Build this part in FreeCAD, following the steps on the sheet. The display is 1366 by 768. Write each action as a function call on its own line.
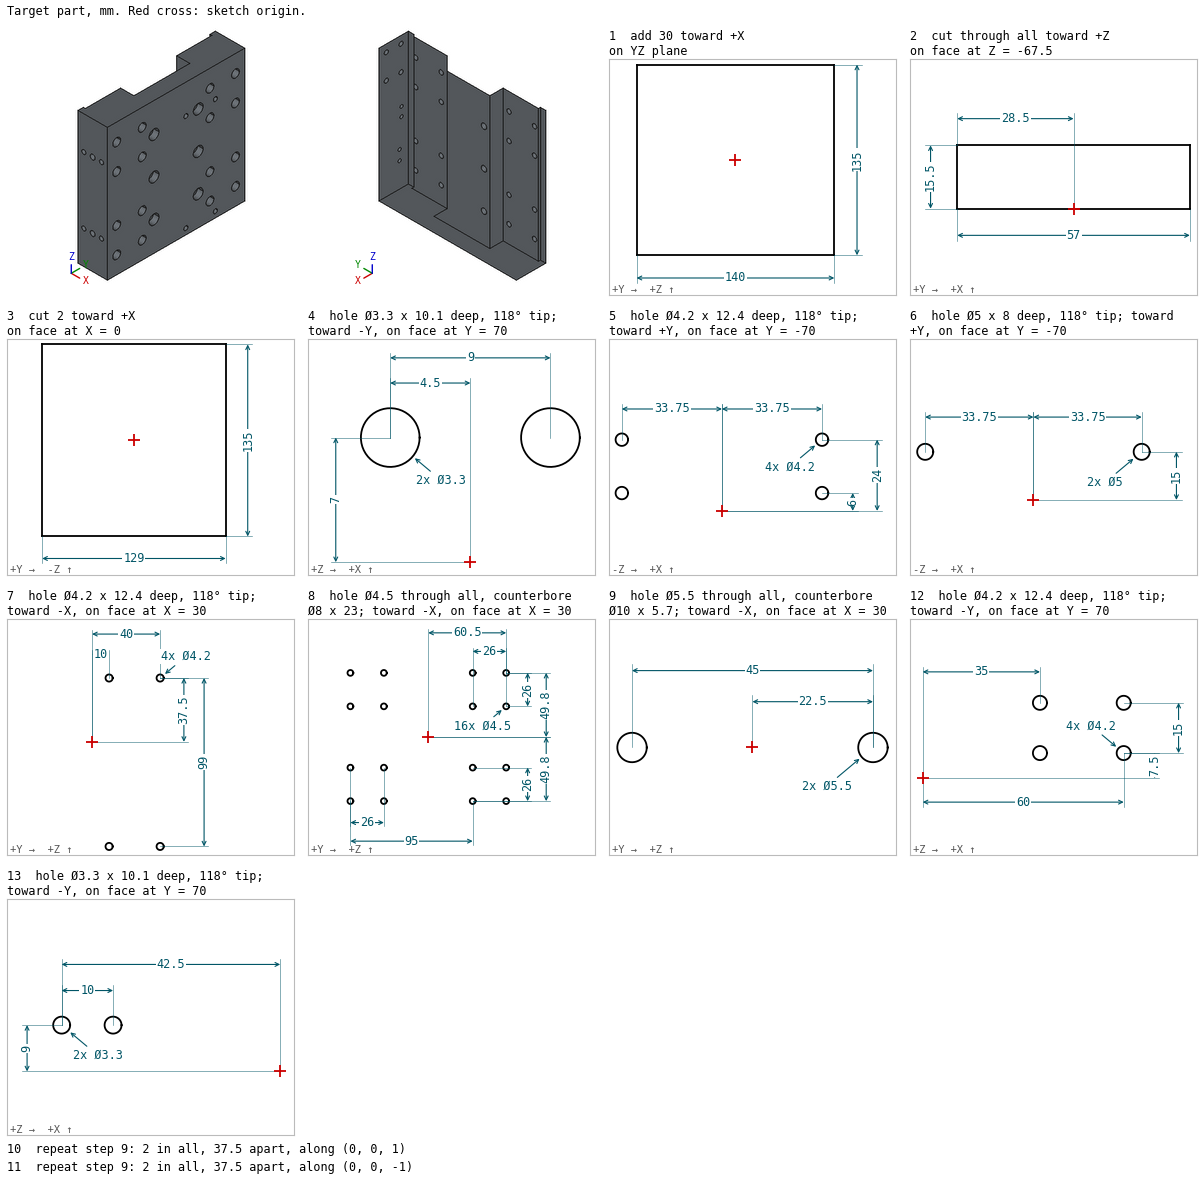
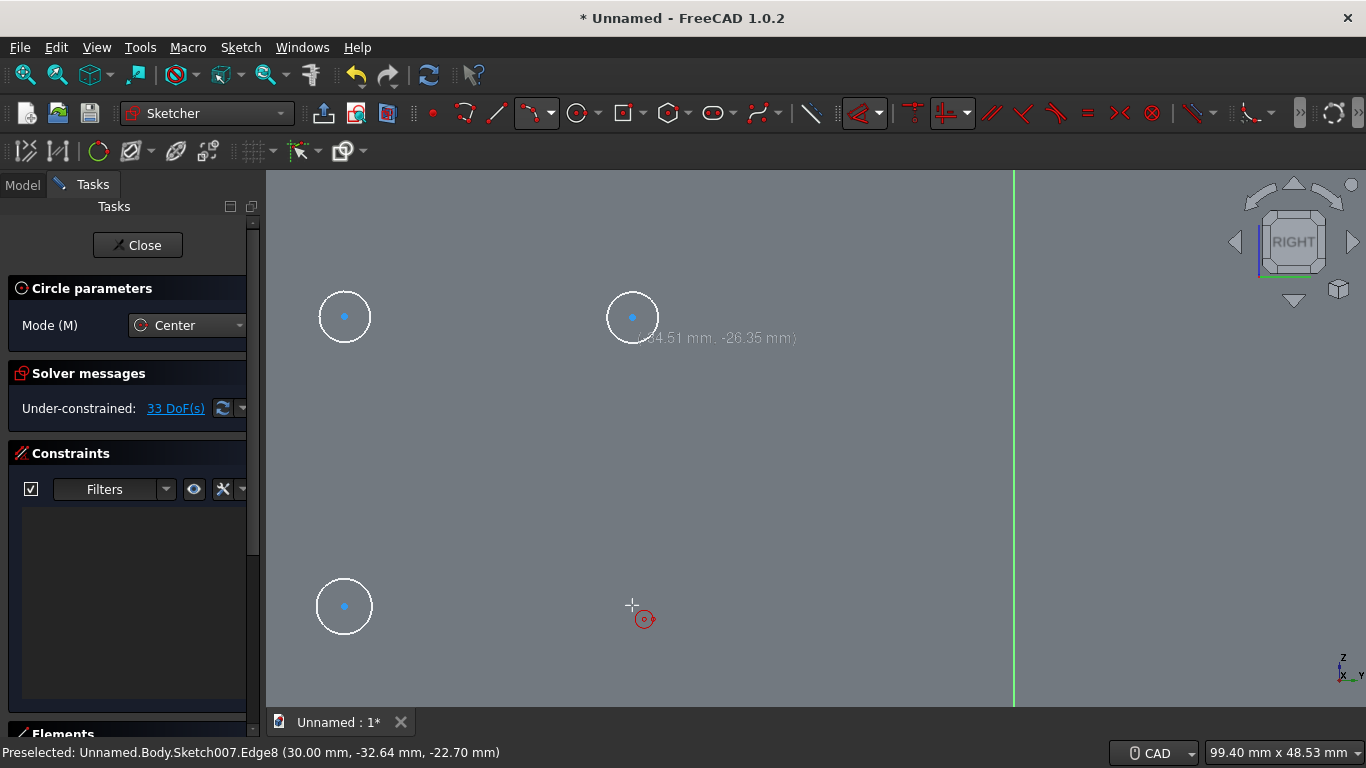
scroll(632, 605, down, 6)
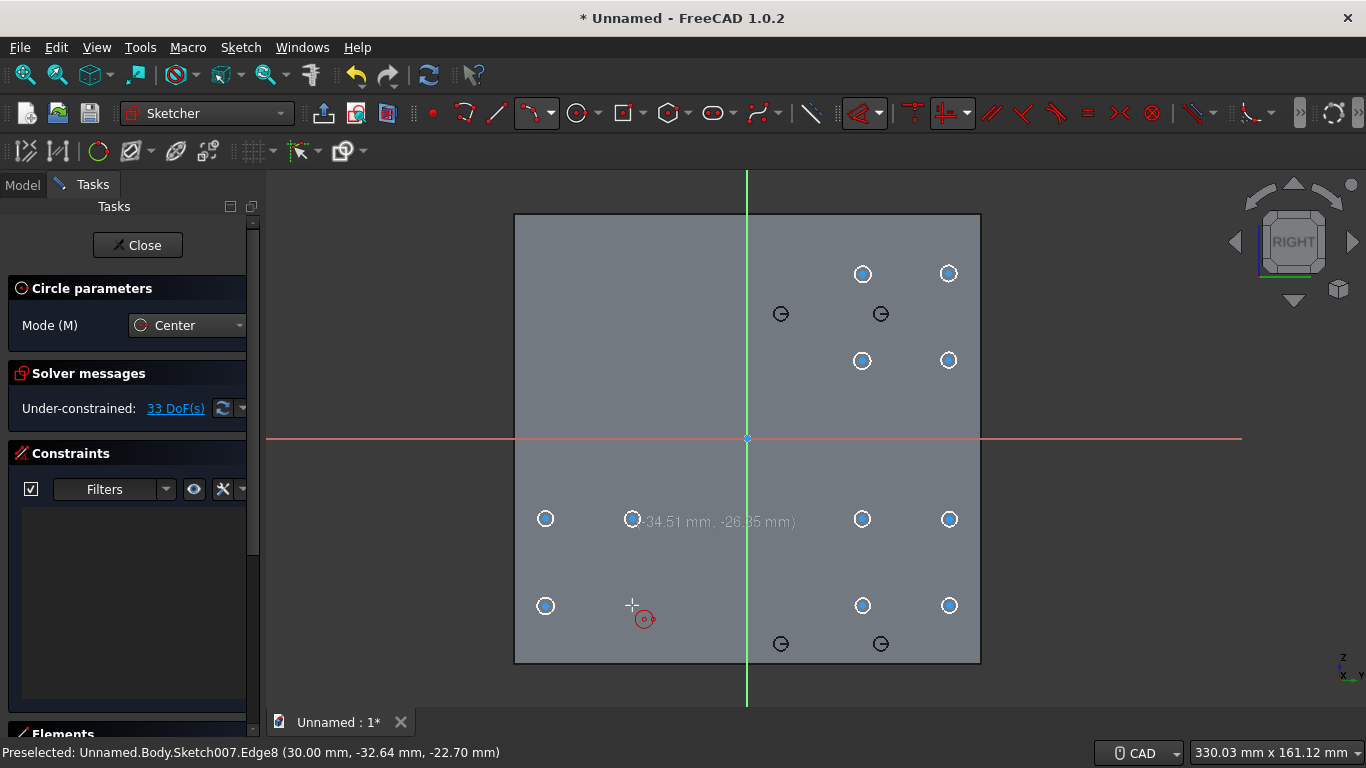
click(632, 605)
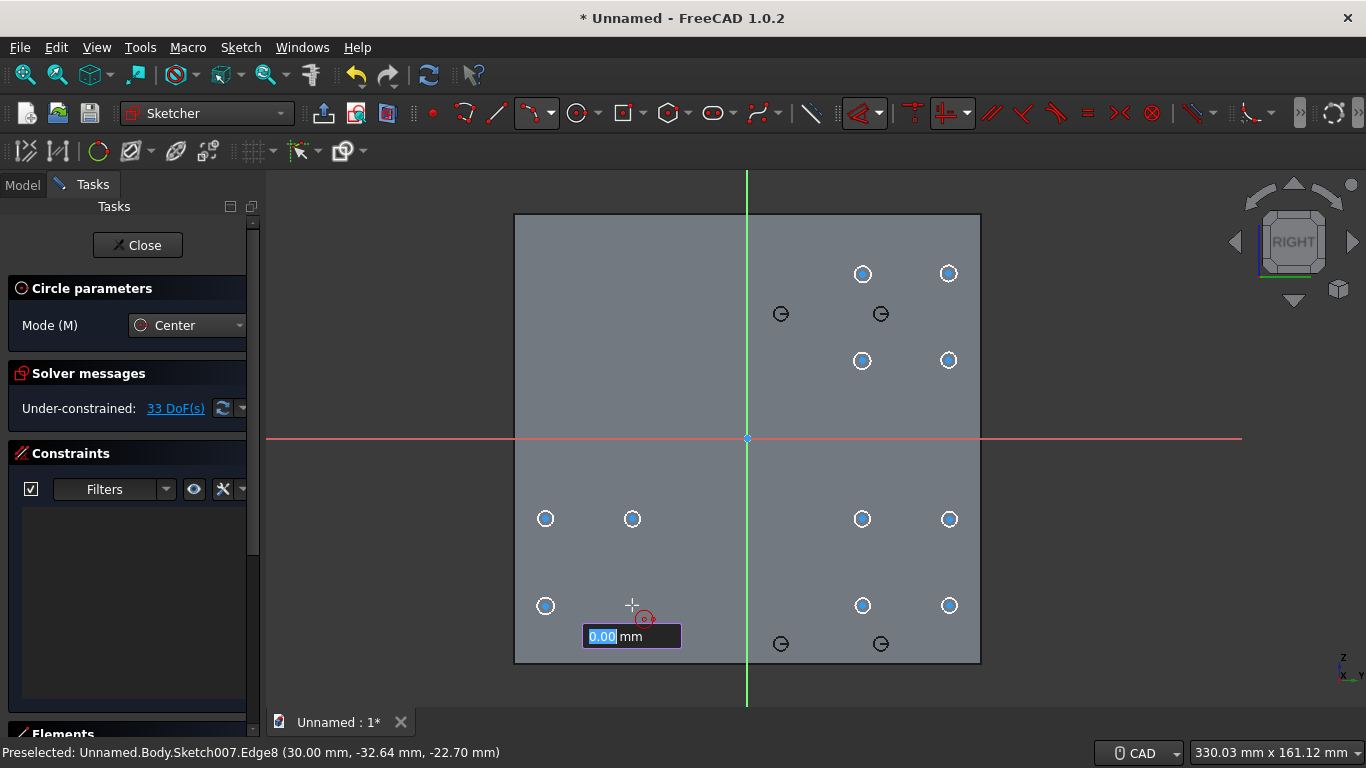
scroll(638, 600, up, 4)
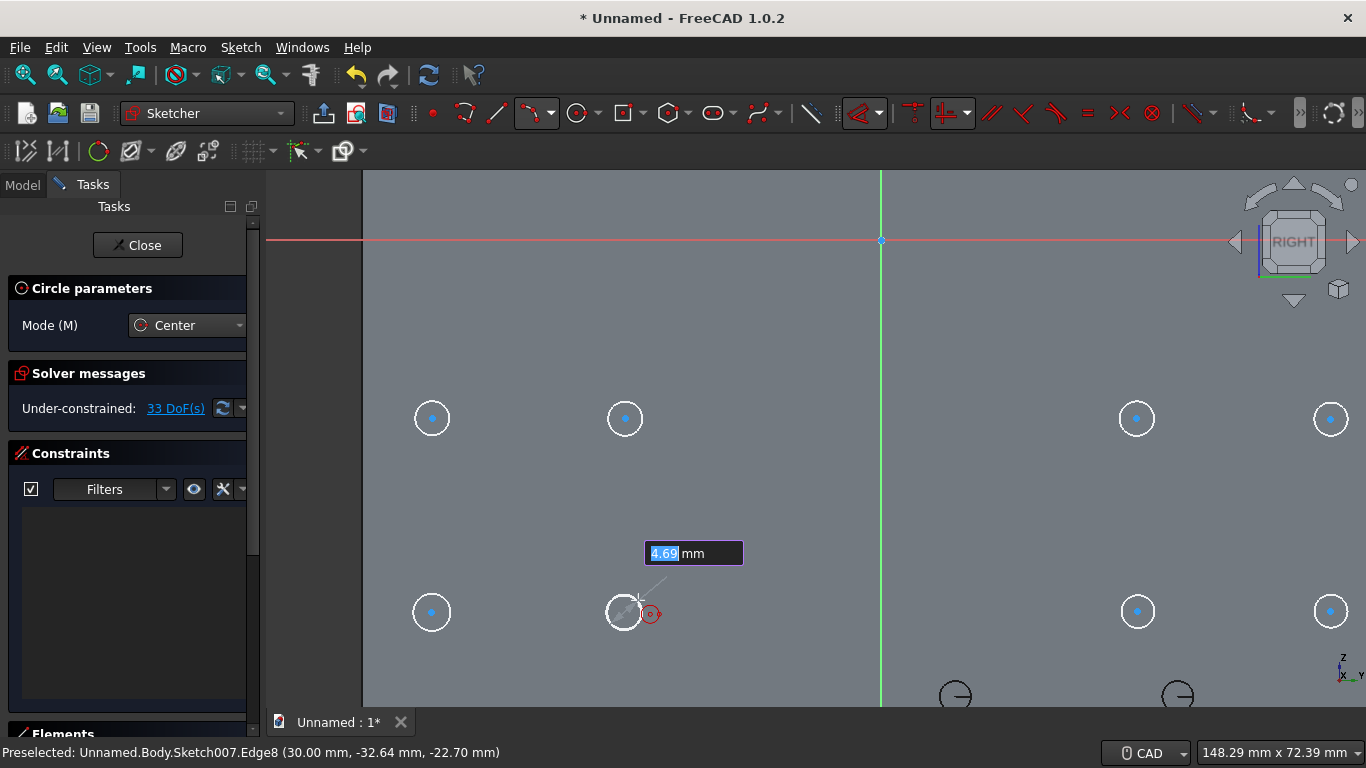
click(637, 598)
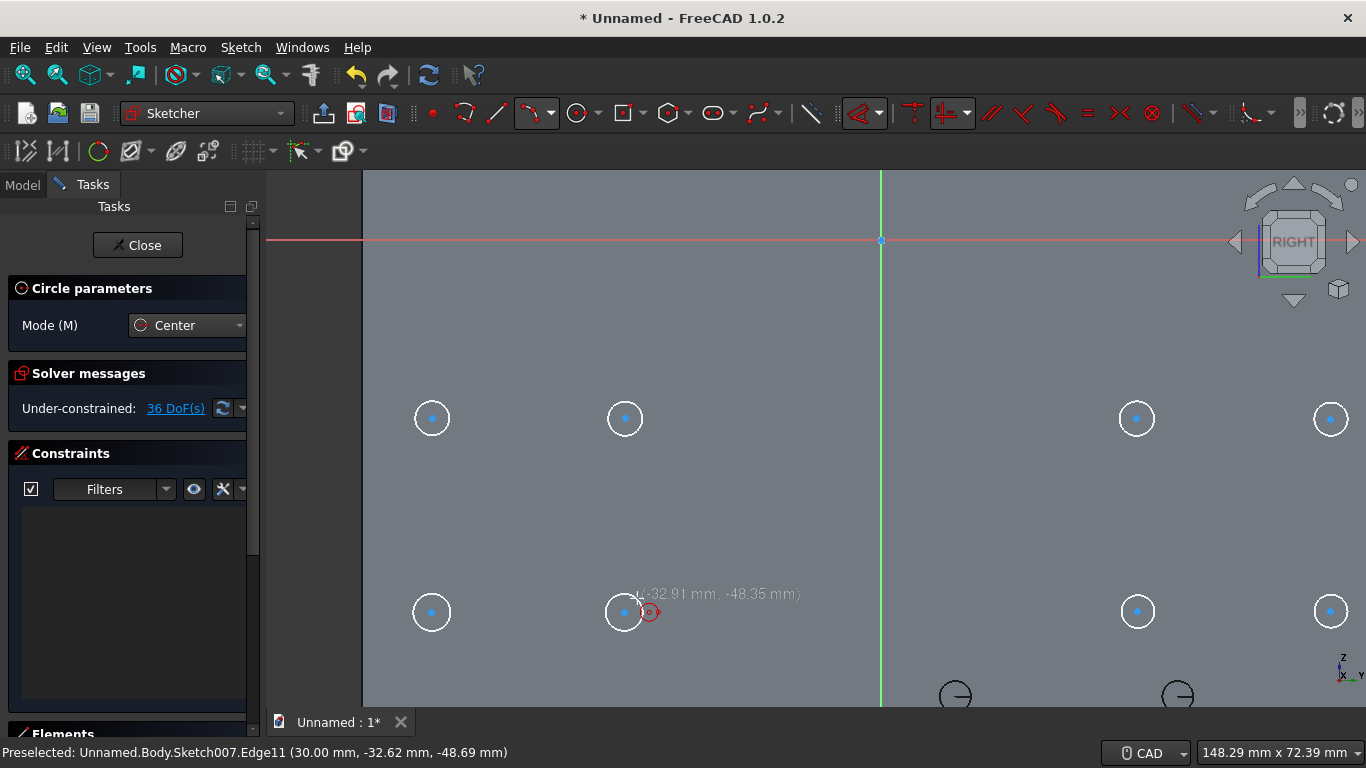
scroll(638, 600, down, 4)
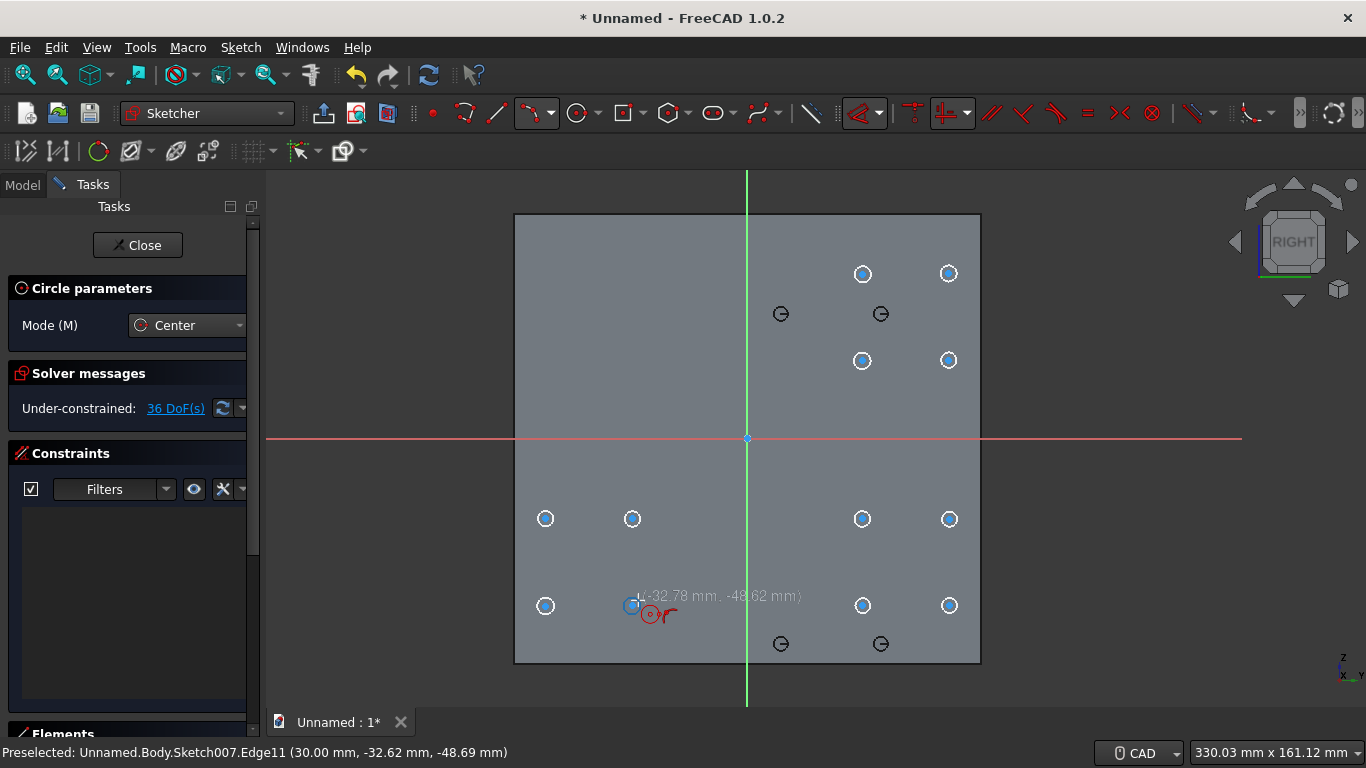
scroll(632, 273, up, 6)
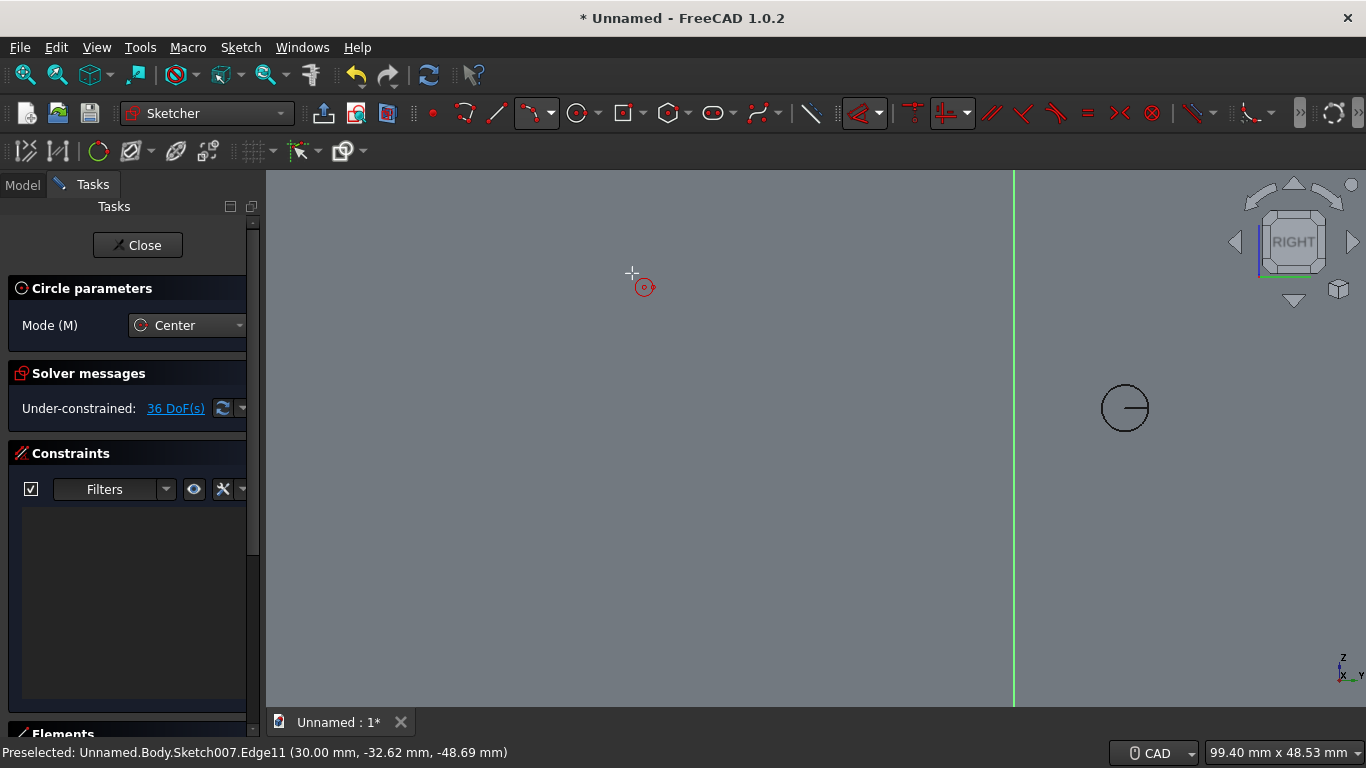
scroll(632, 273, down, 6)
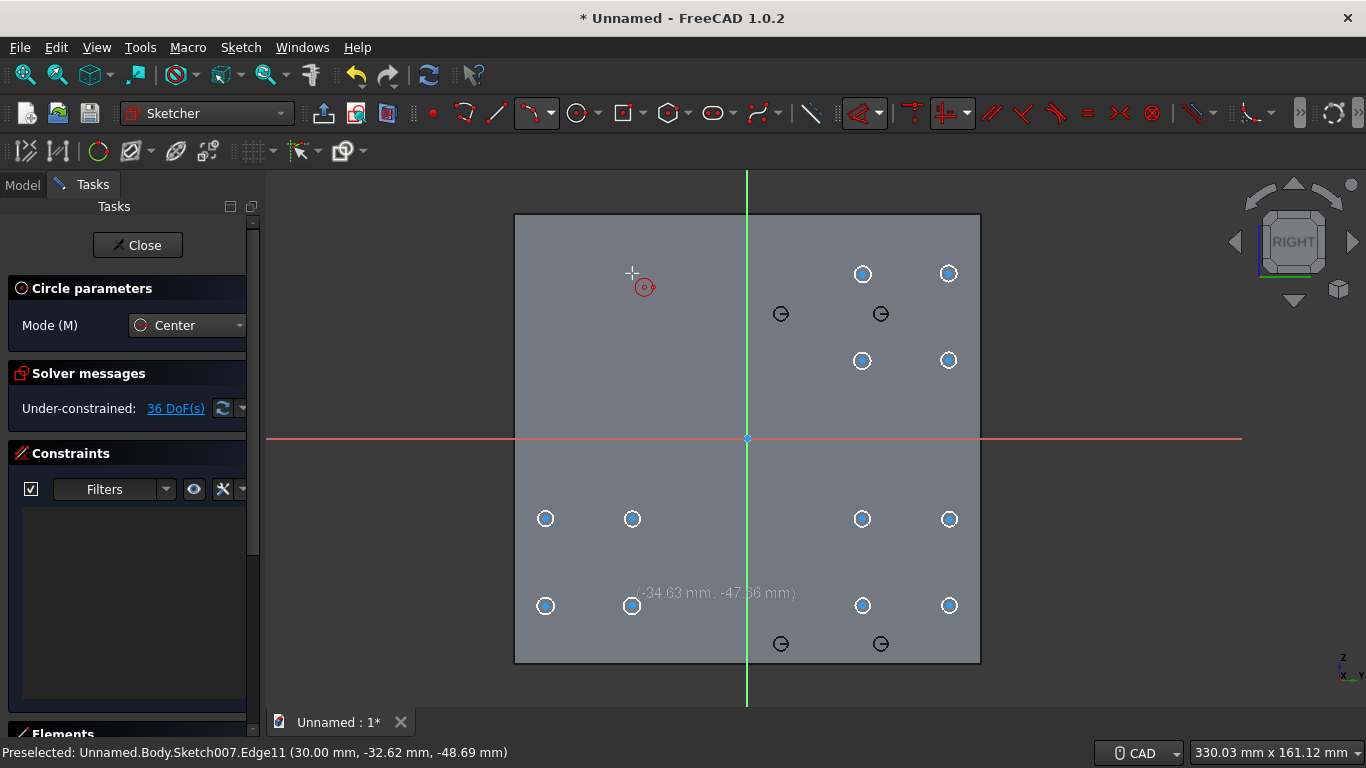
click(632, 273)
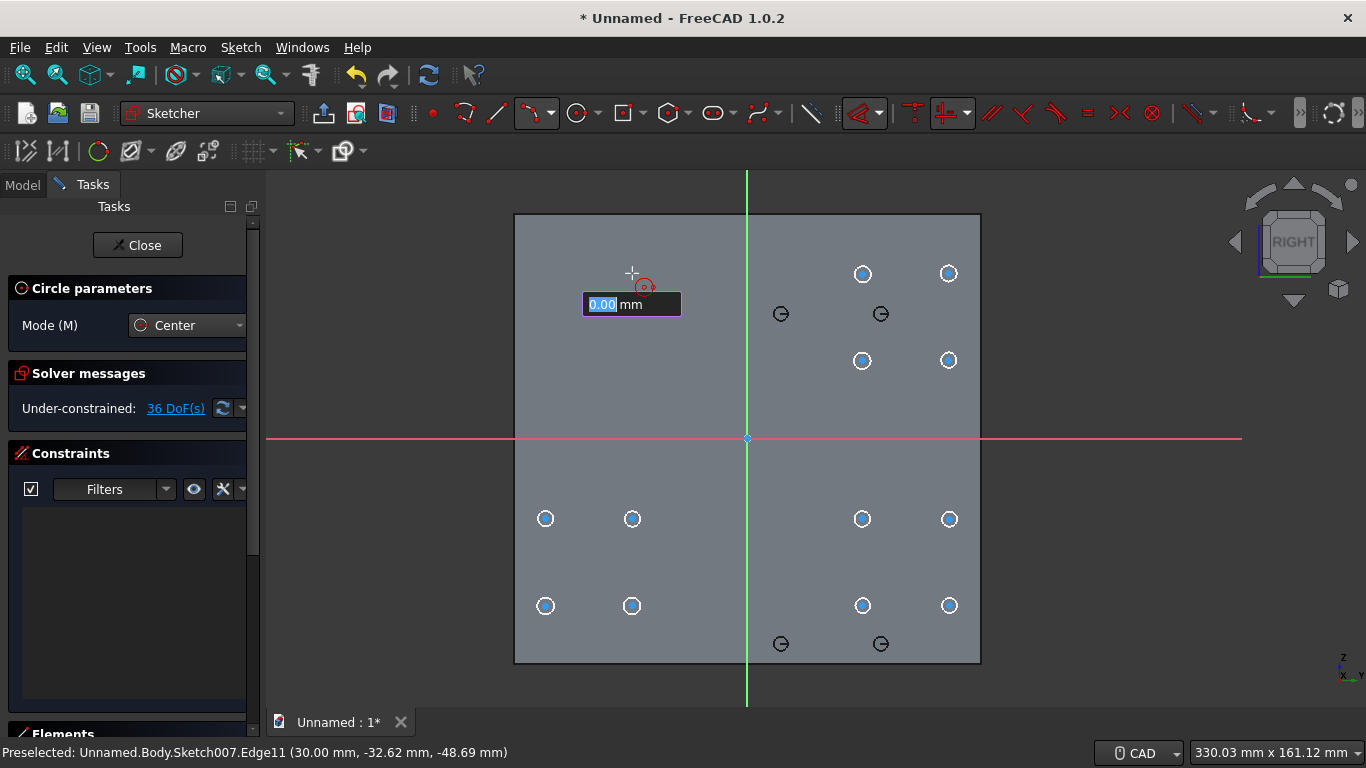
scroll(638, 268, up, 4)